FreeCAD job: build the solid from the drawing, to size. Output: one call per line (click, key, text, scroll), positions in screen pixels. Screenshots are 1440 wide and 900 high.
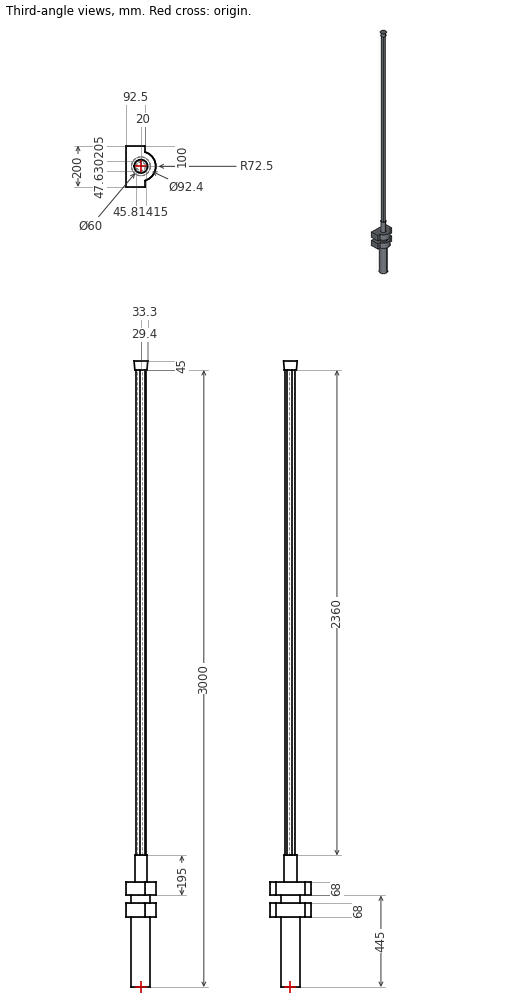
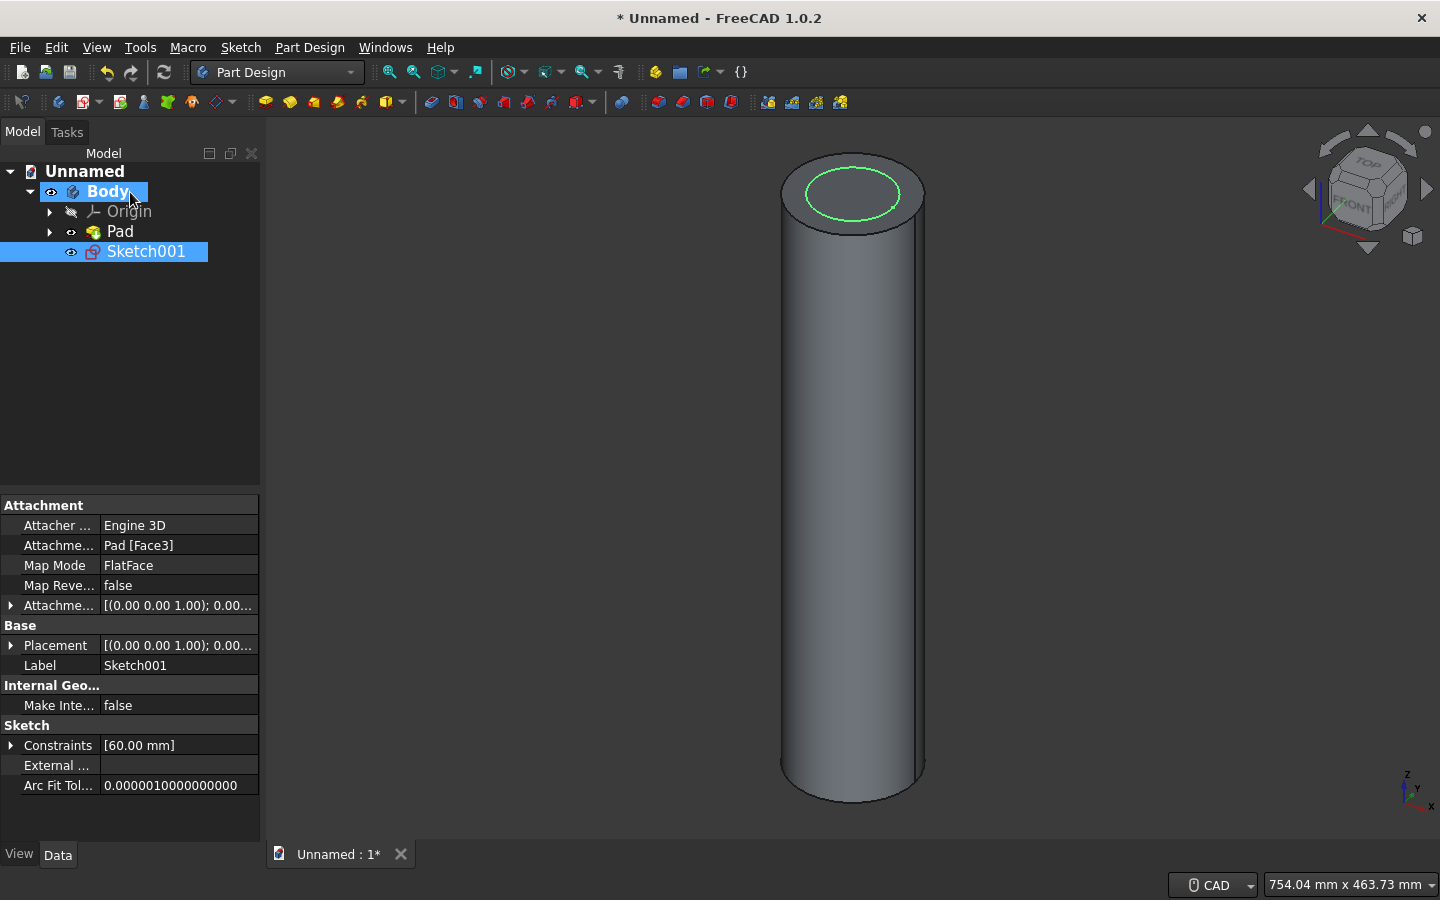
click(266, 102)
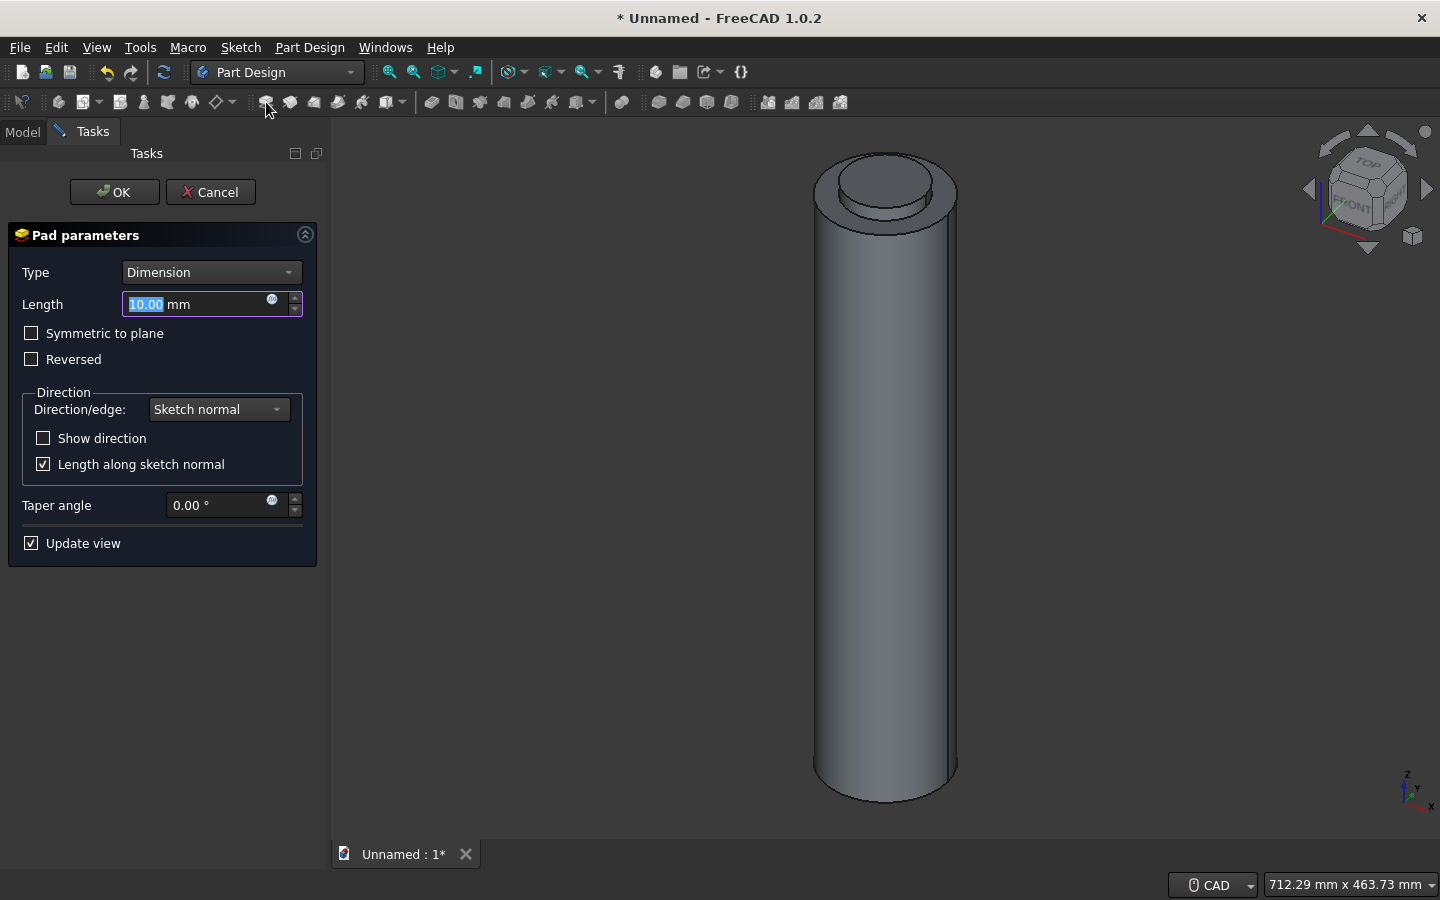
text(195)
key(Tab)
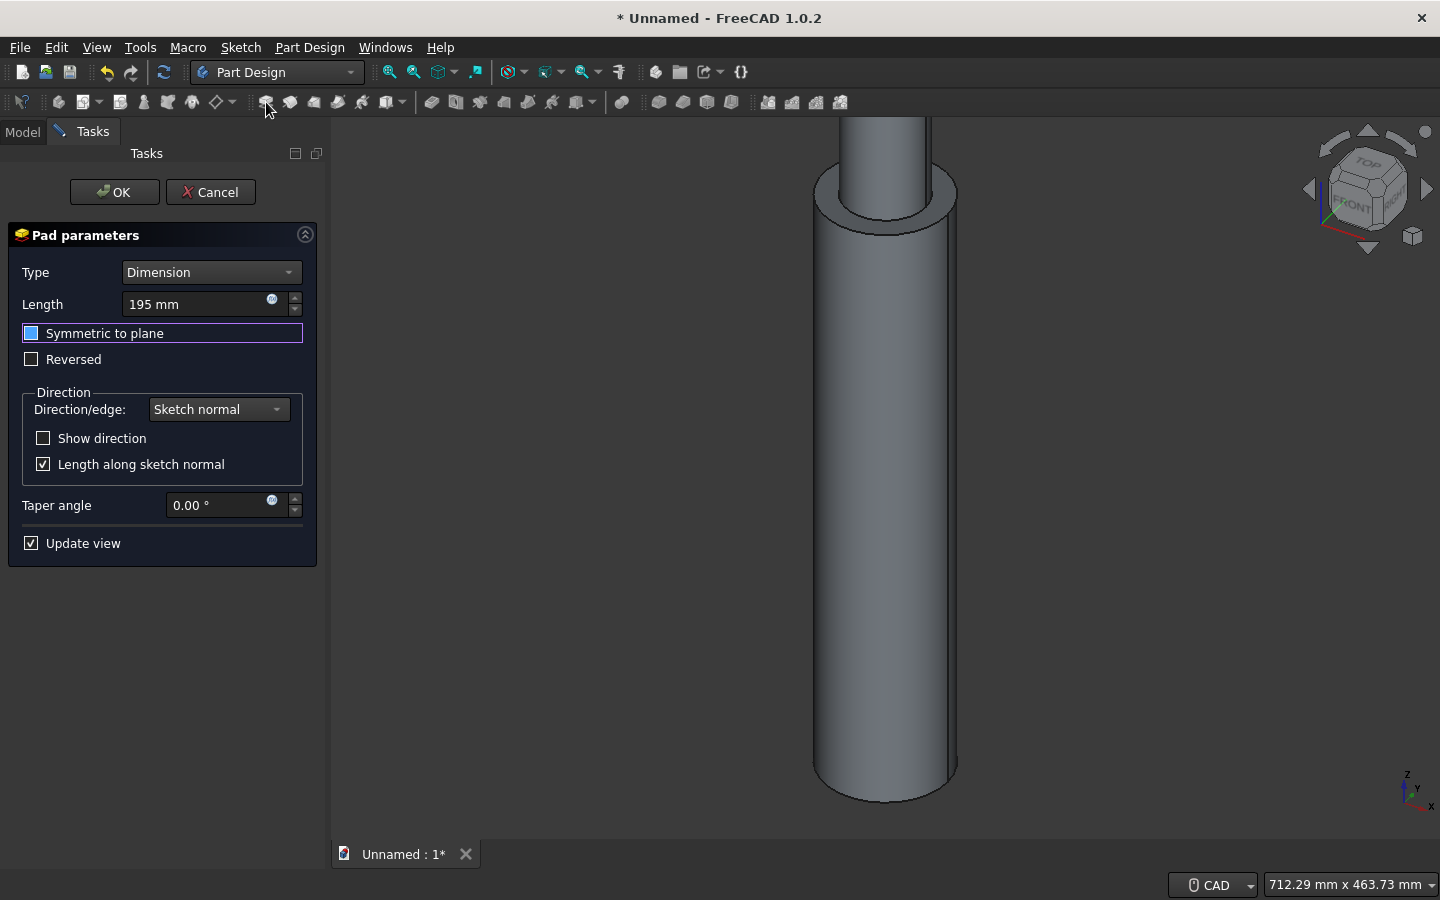
click(115, 192)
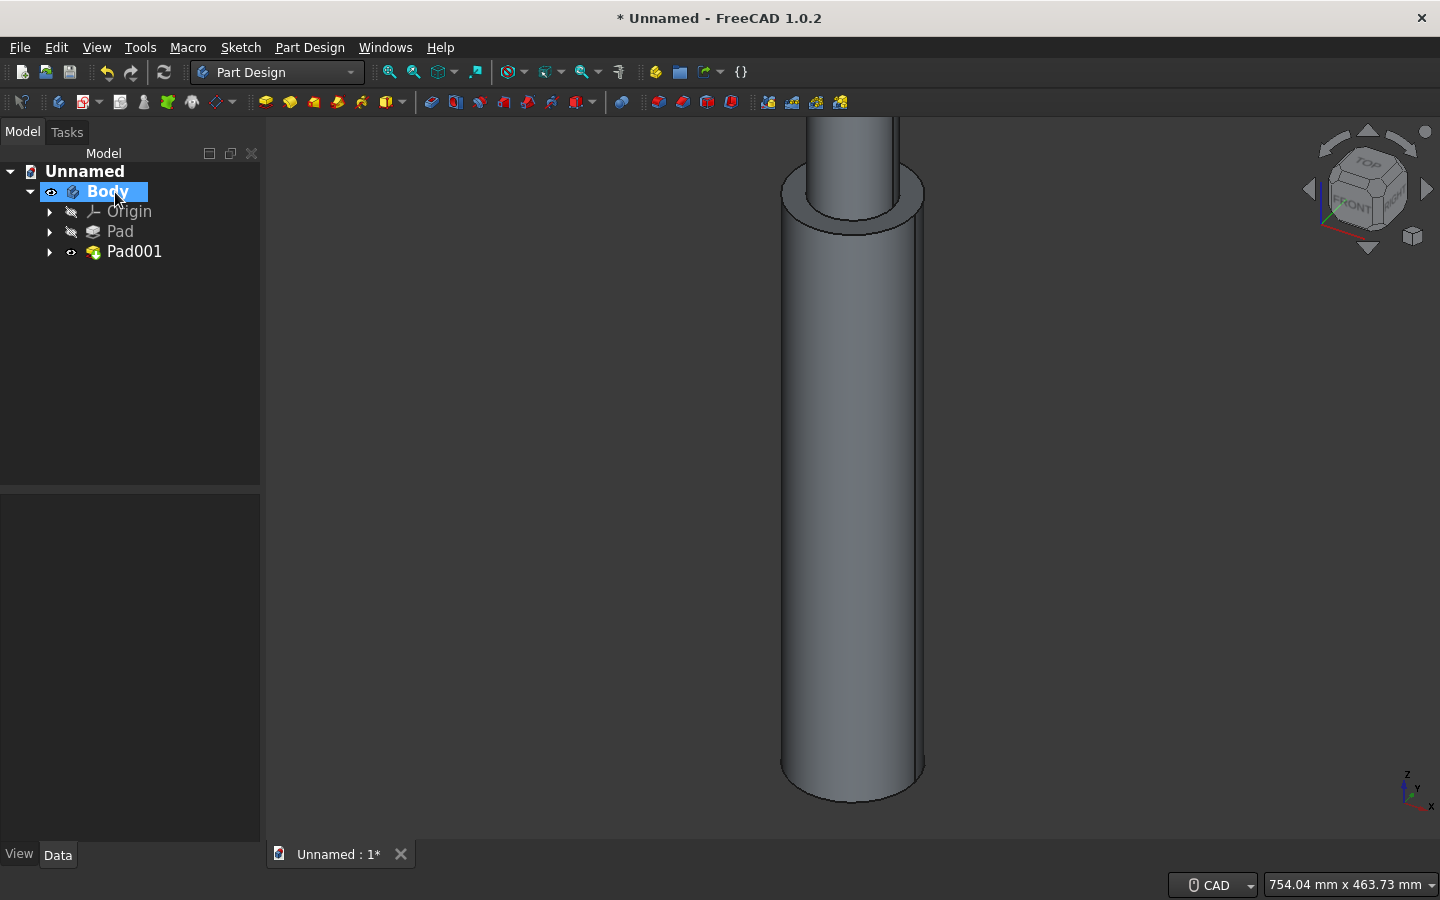
key(v)
key(f)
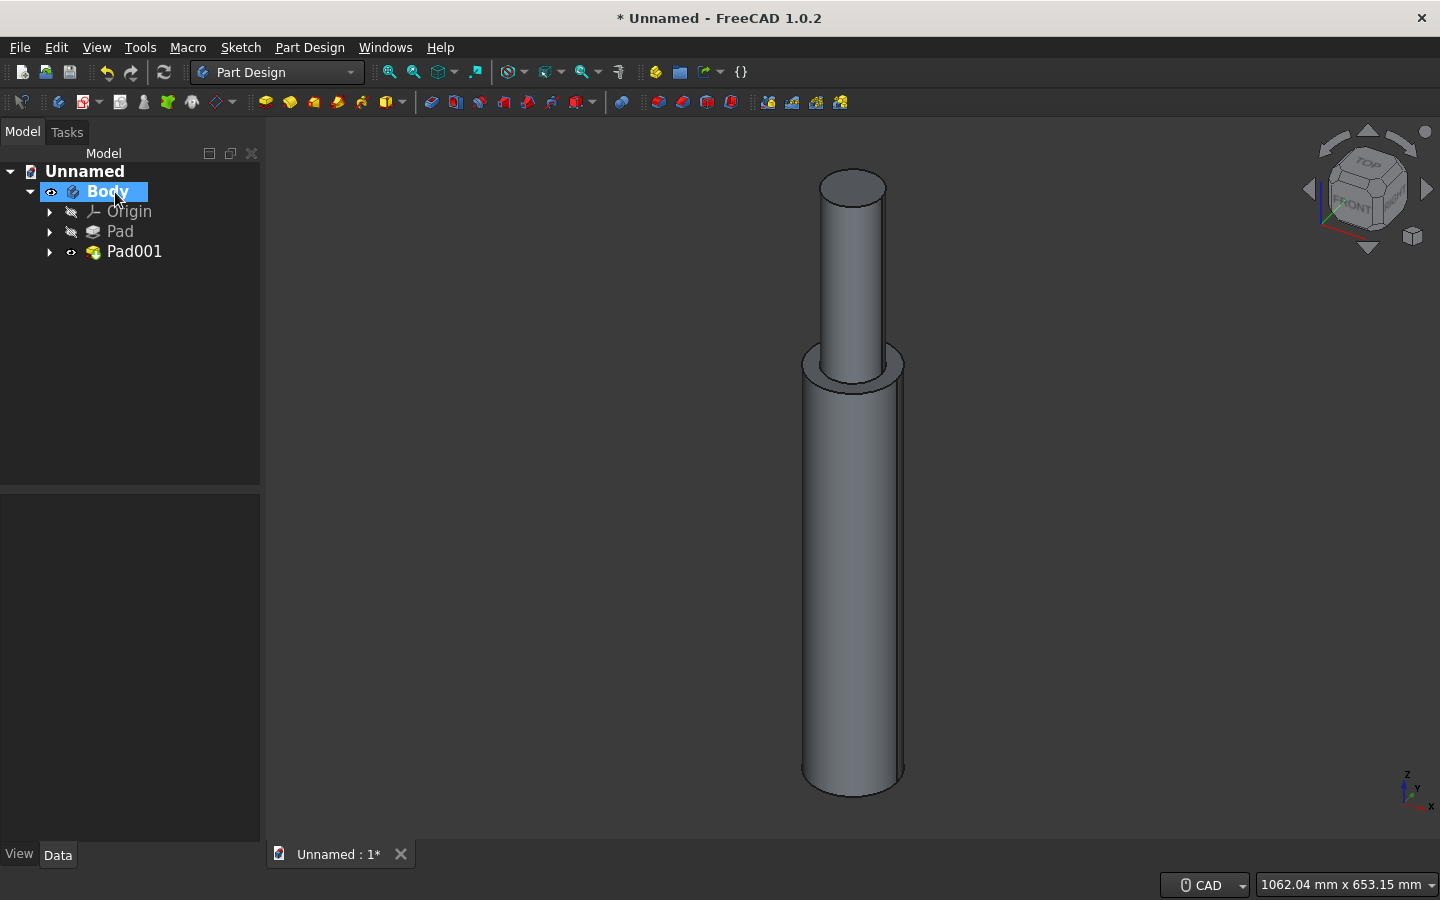
click(853, 187)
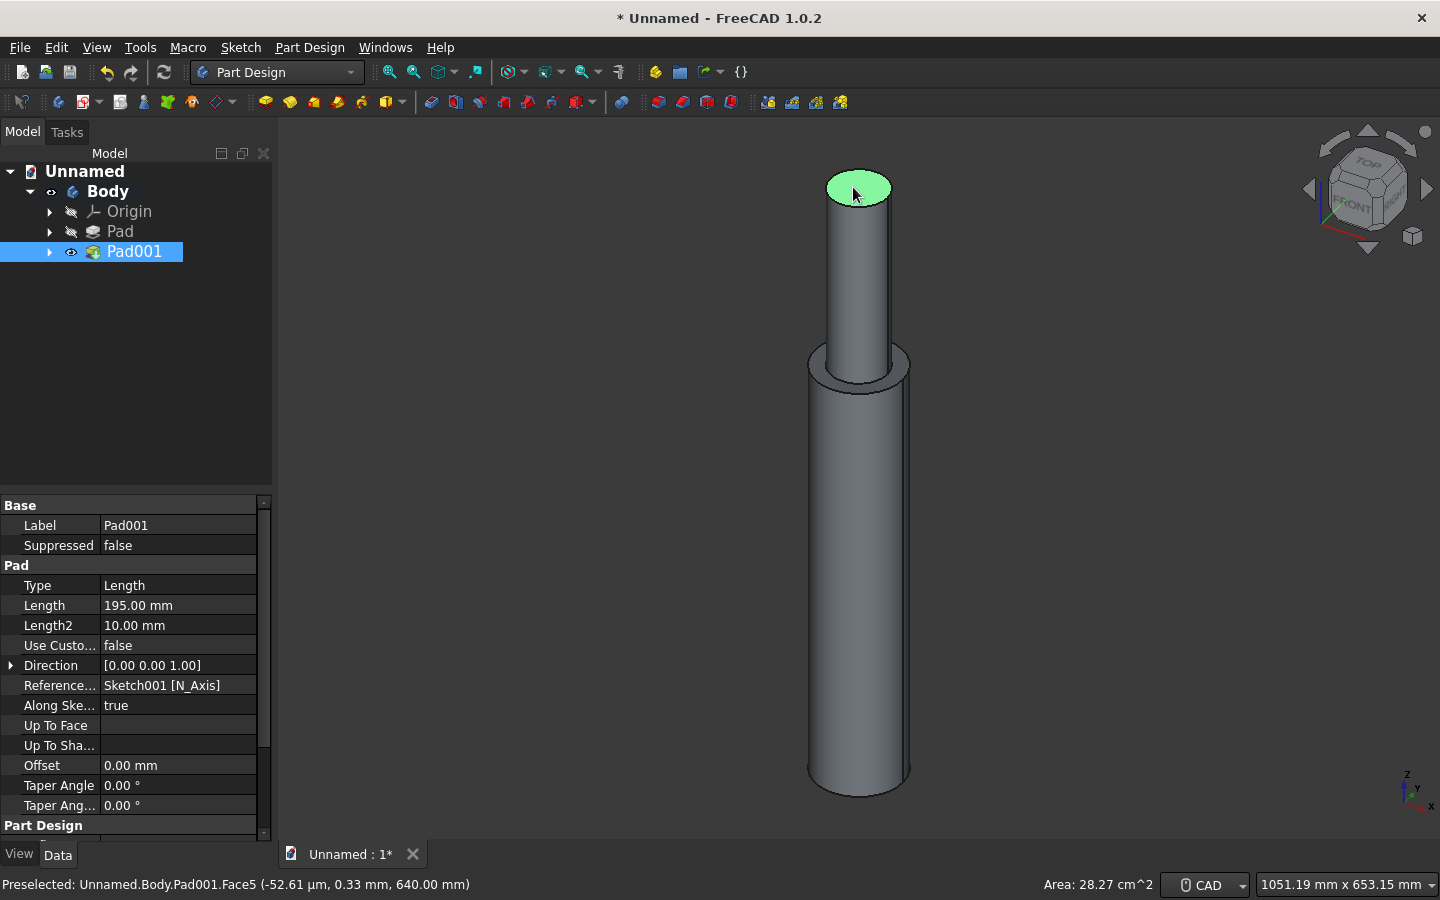
click(84, 102)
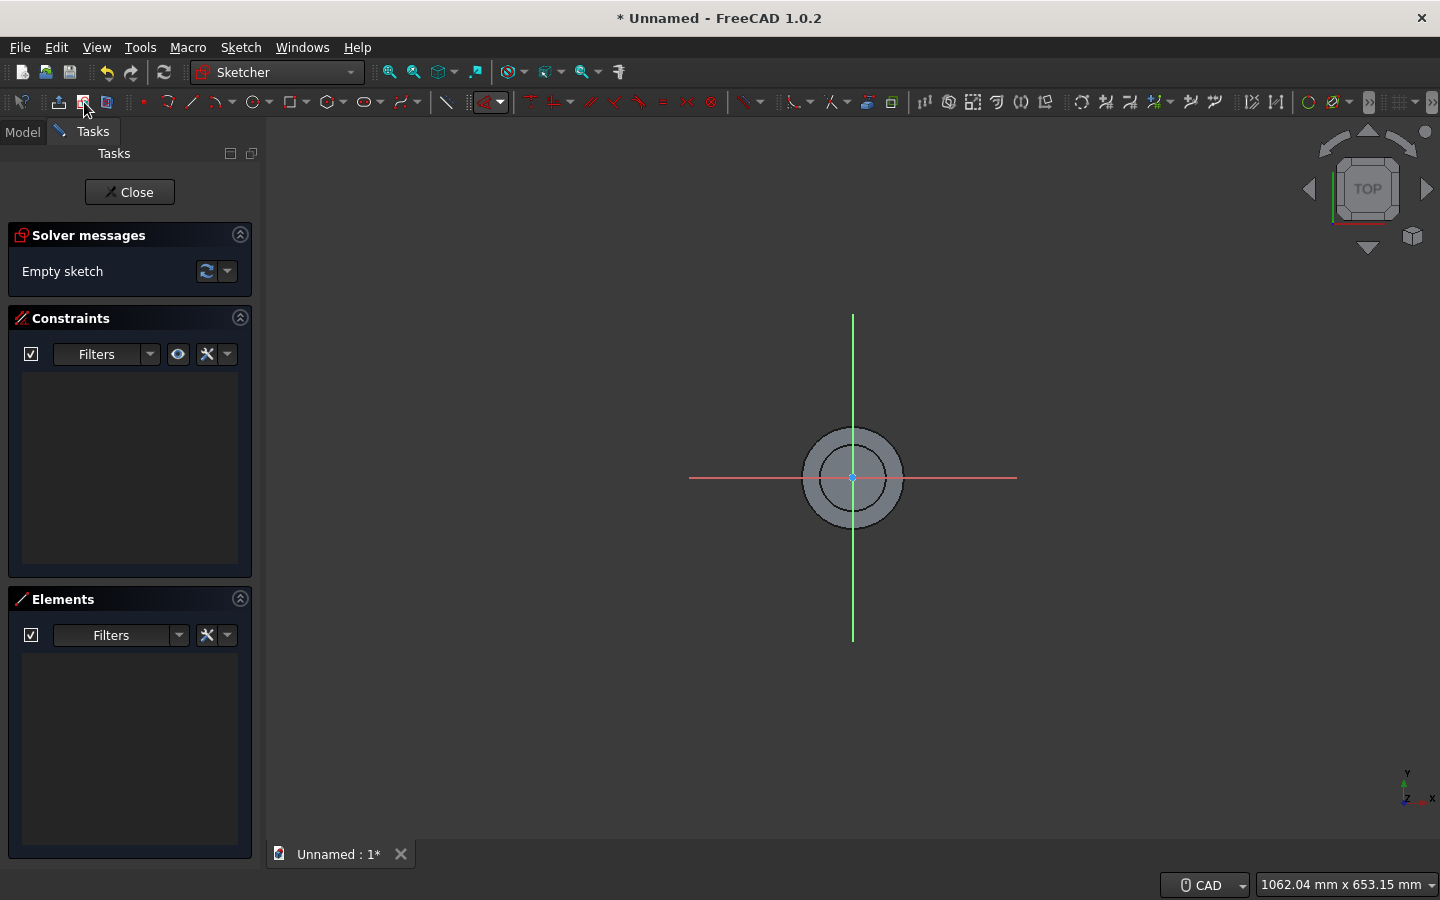
scroll(861, 478, up, 11)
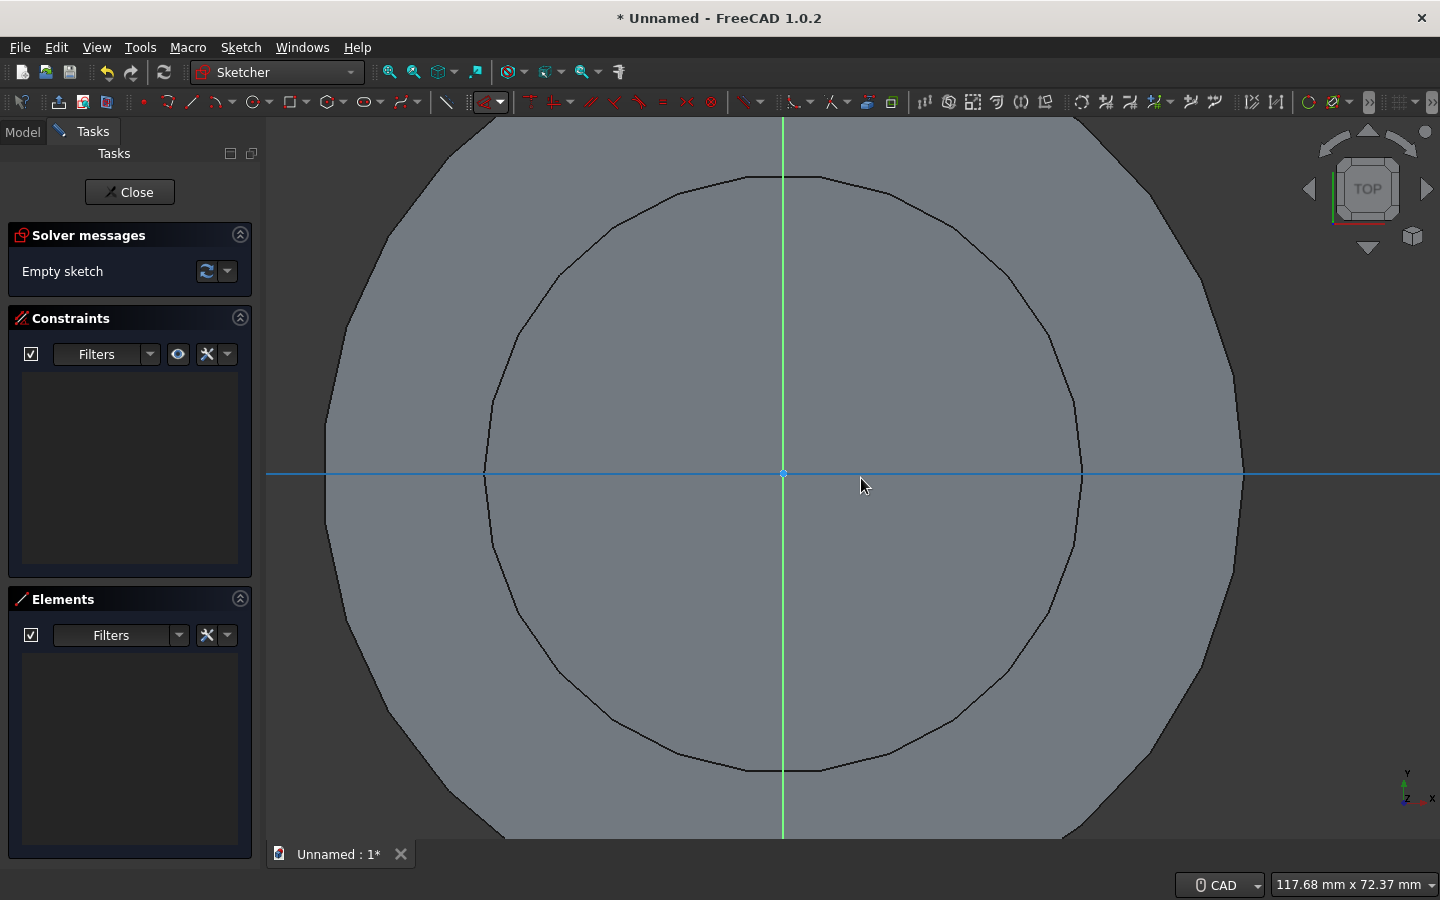
click(328, 102)